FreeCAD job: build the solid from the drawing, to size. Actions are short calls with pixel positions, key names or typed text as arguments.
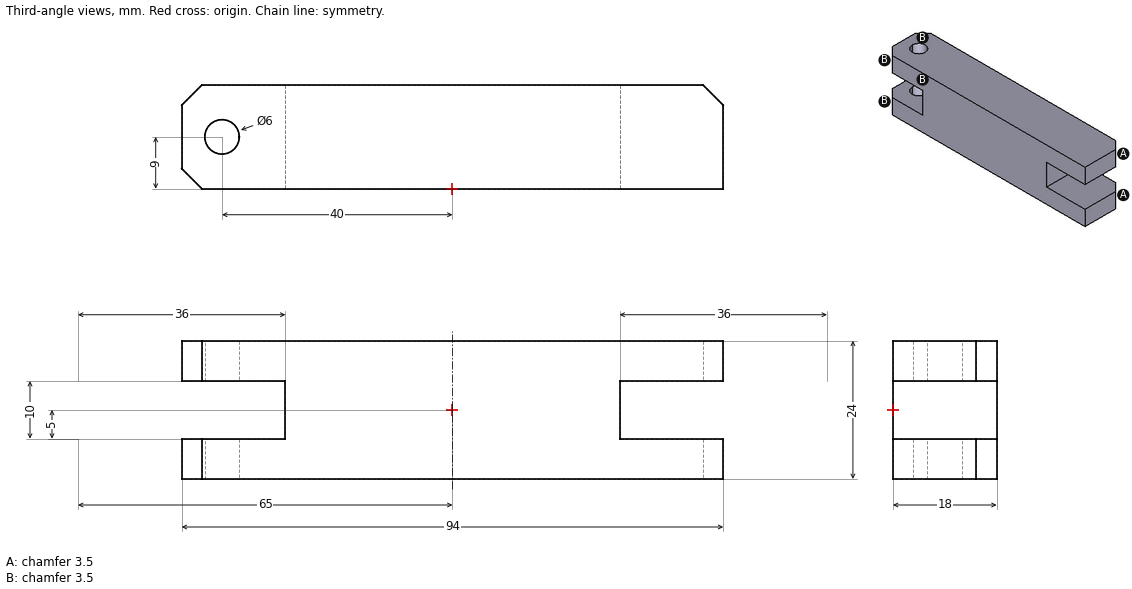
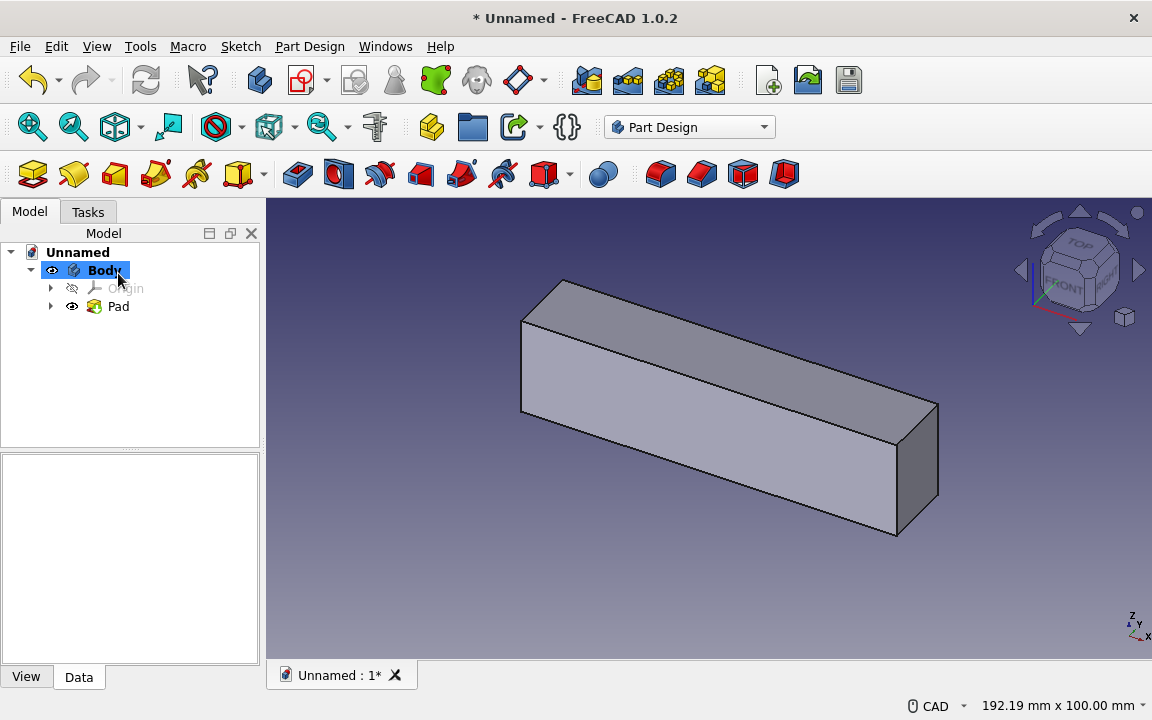
key(4)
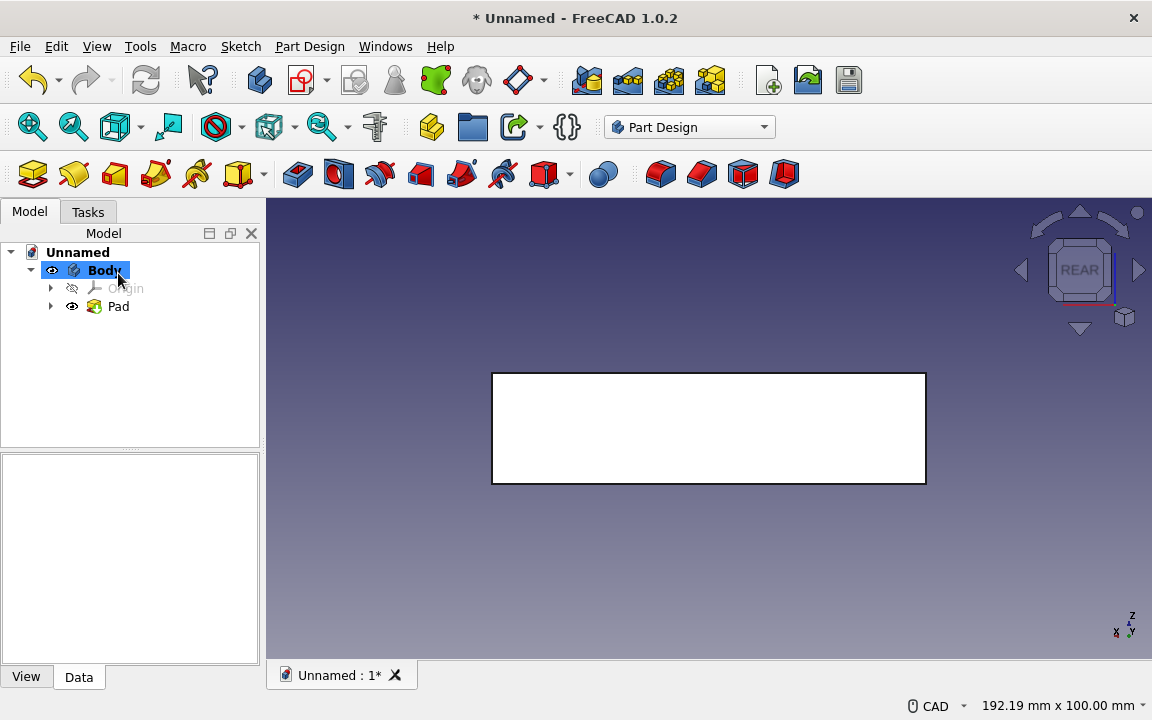
click(585, 427)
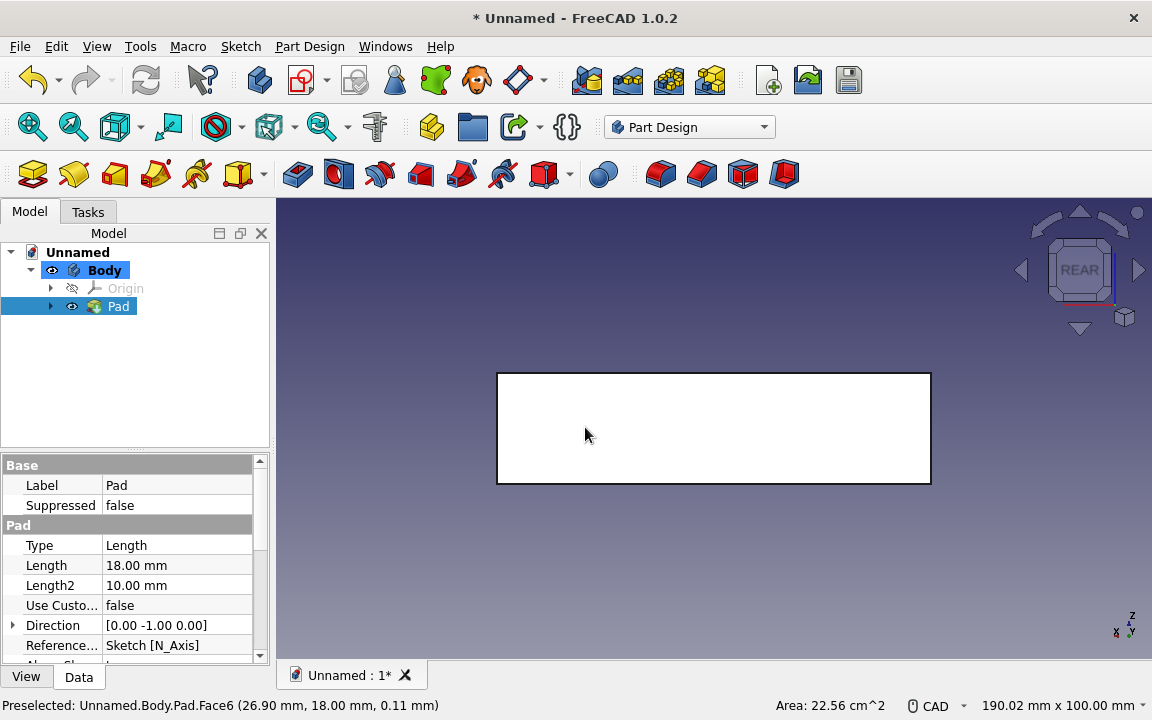
click(300, 80)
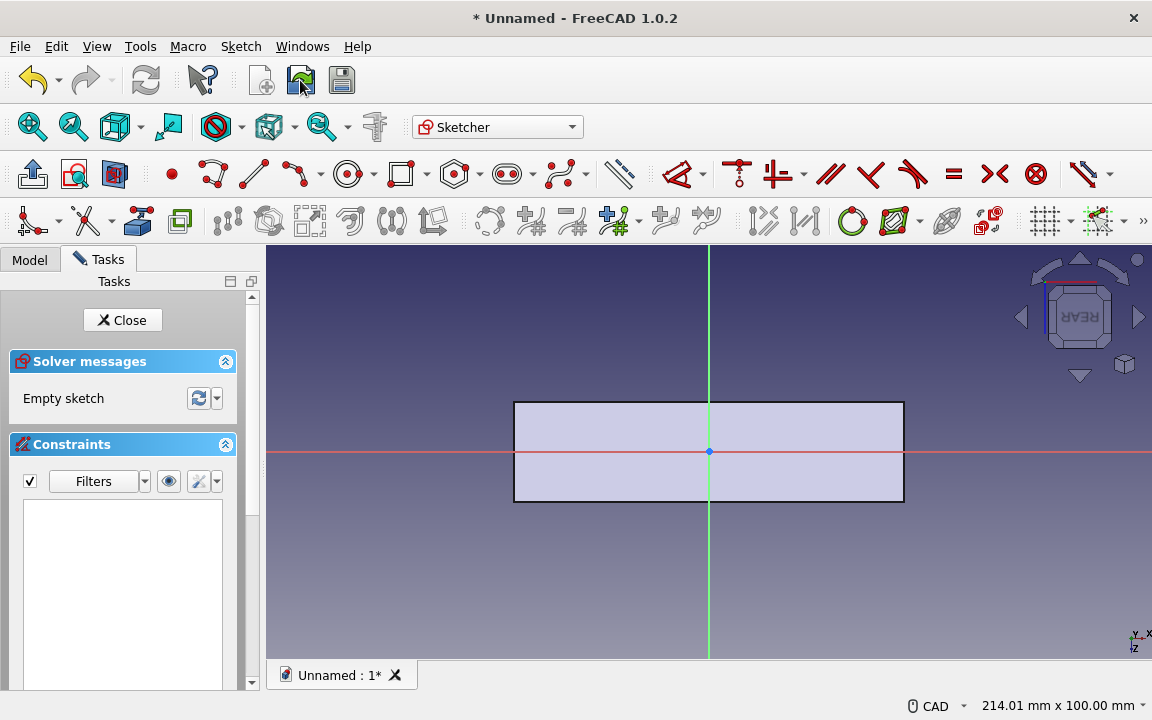
scroll(331, 452, down, 1)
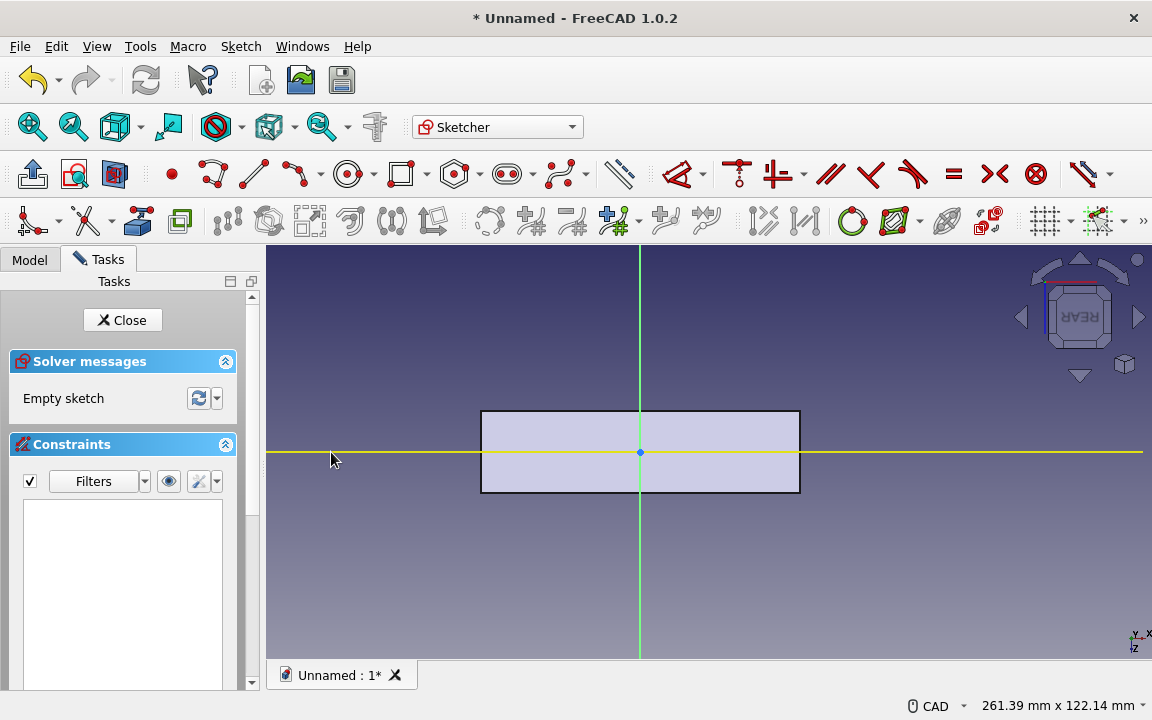
key(g)
key(r)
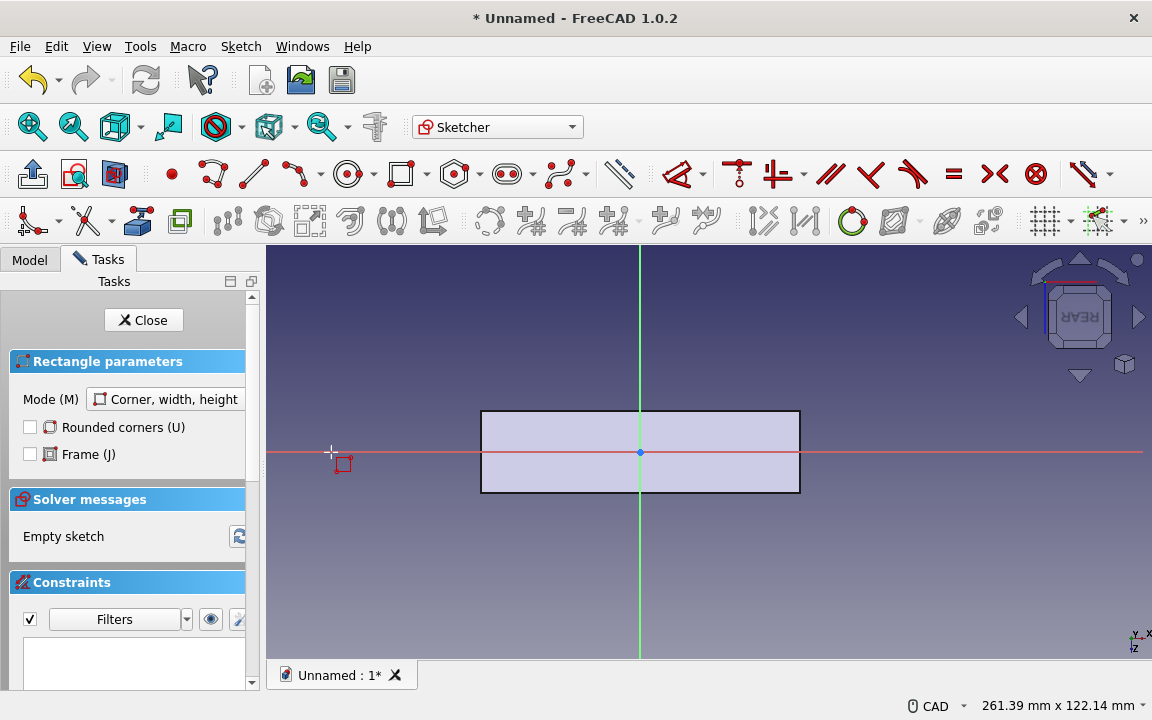
click(420, 435)
move(542, 469)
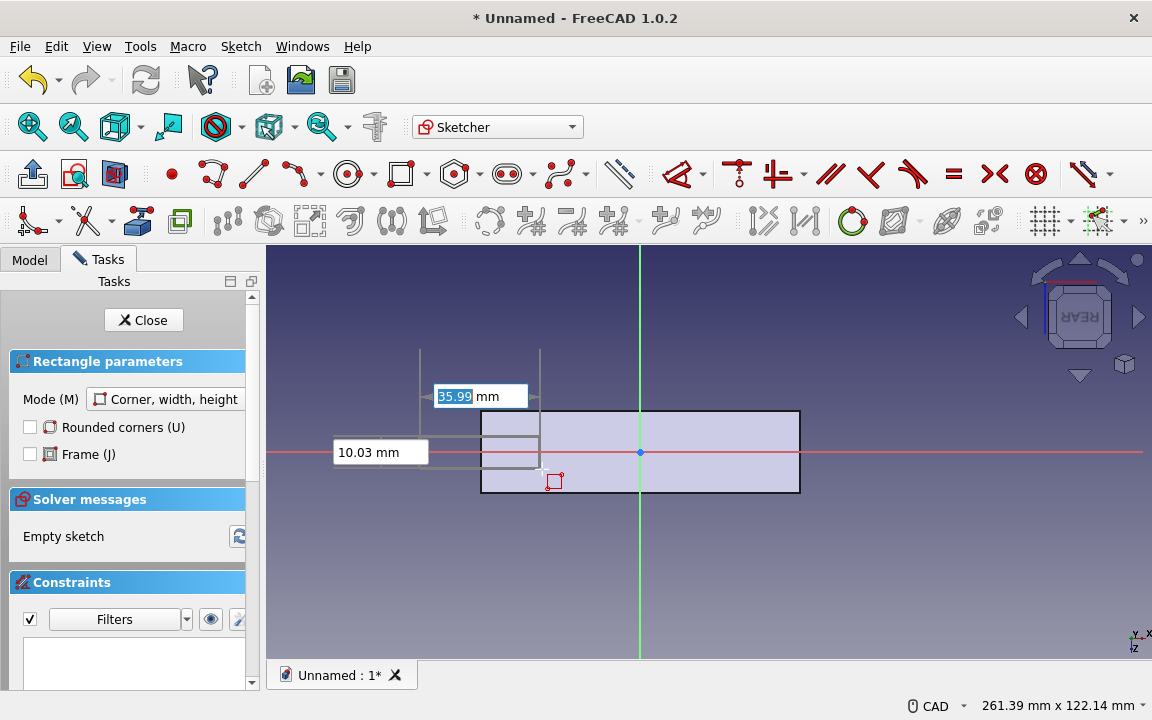
text(36)
key(Tab)
text(10)
key(Return)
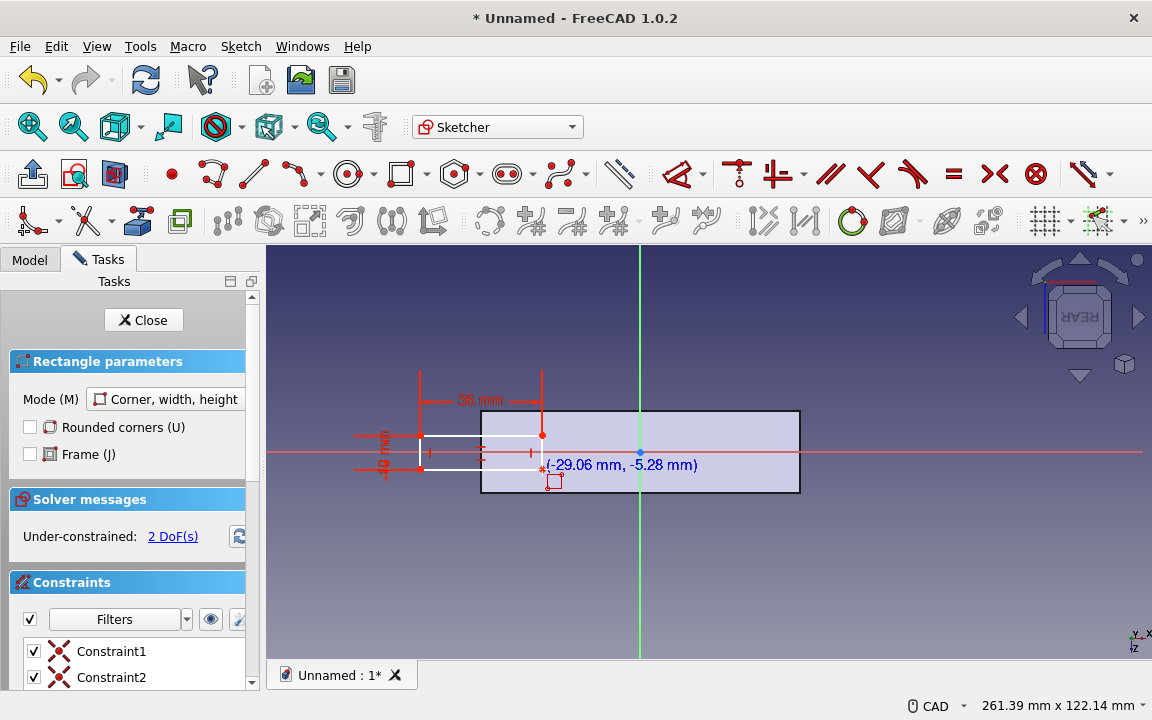
click(739, 435)
move(861, 469)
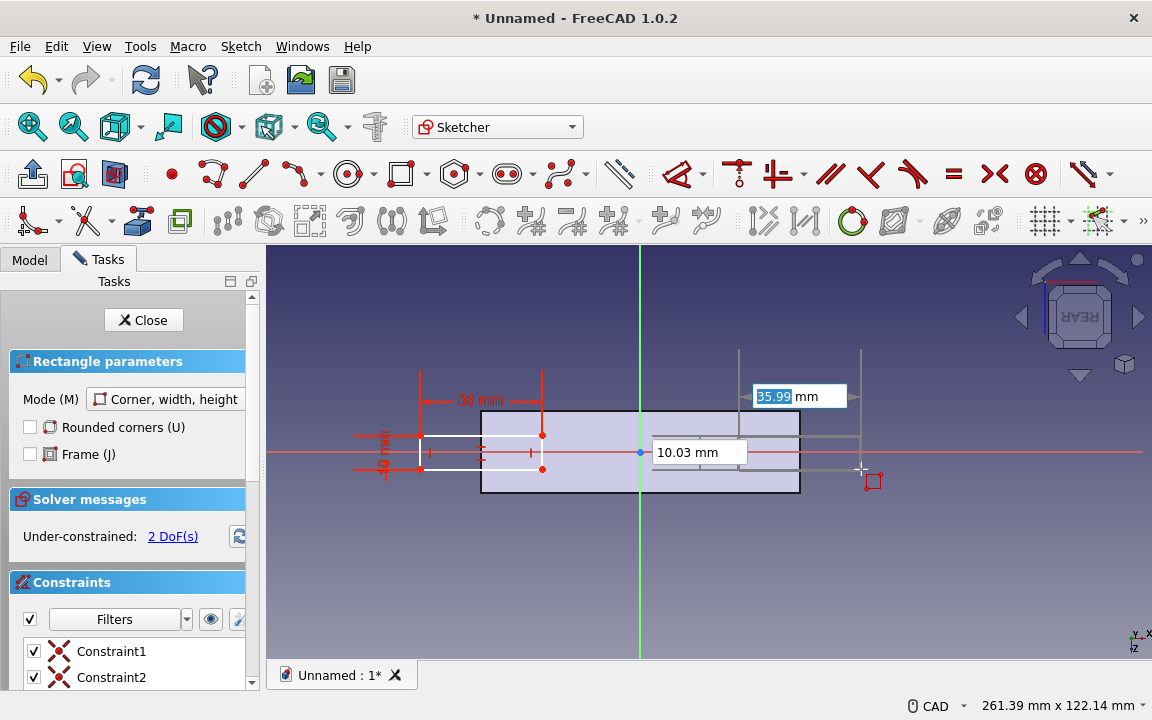
text(36)
key(Tab)
text(10)
key(Return)
key(Escape)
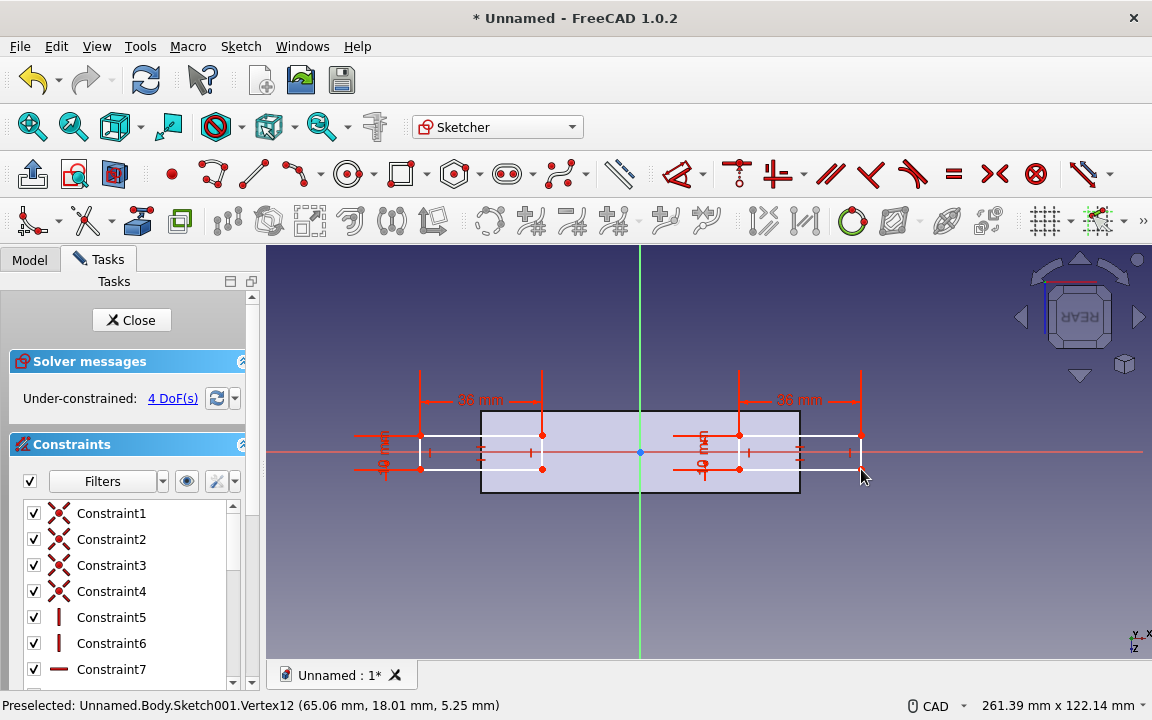
click(542, 436)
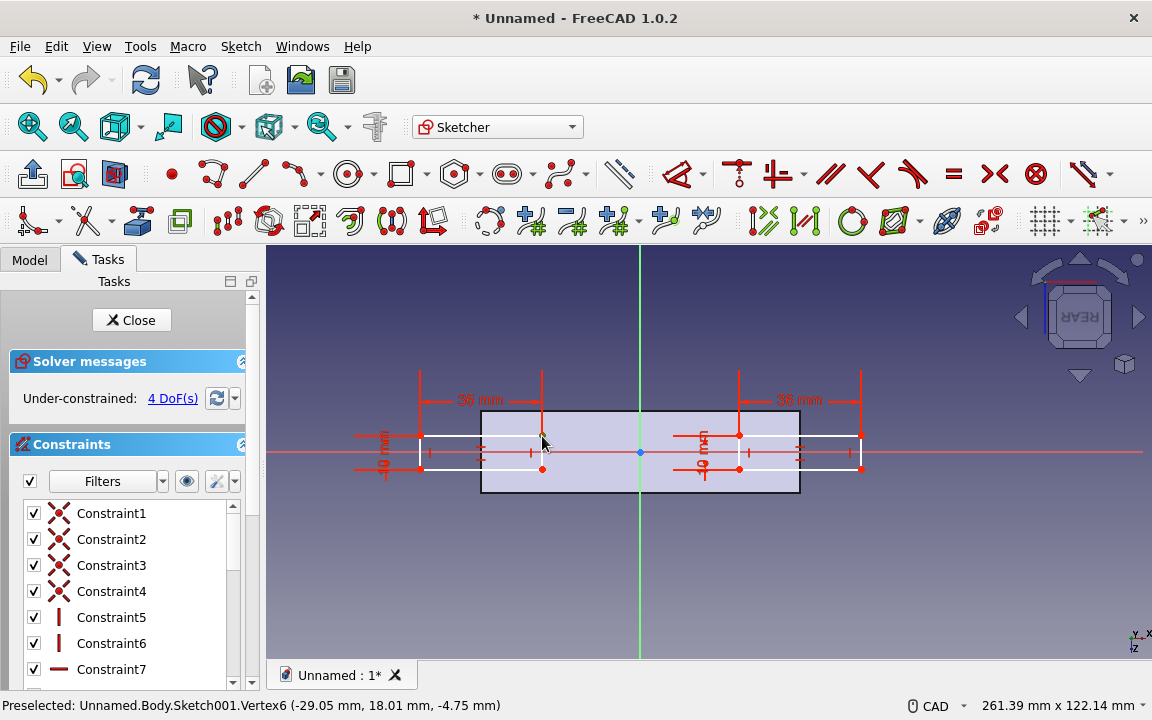
click(739, 436)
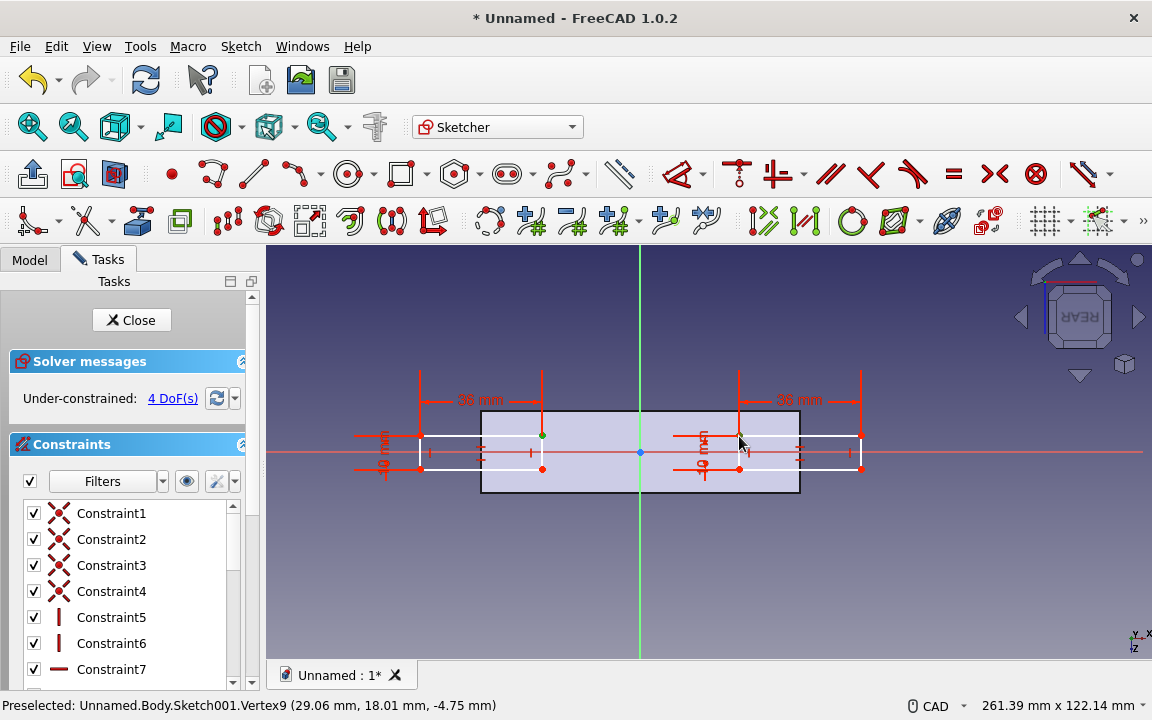
click(640, 605)